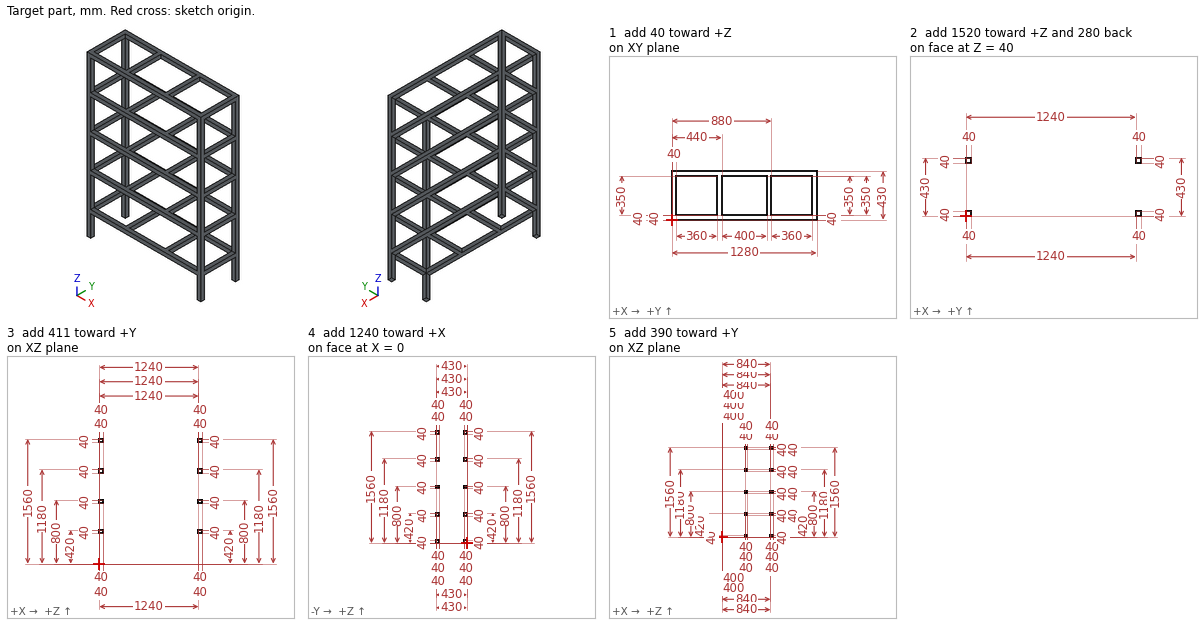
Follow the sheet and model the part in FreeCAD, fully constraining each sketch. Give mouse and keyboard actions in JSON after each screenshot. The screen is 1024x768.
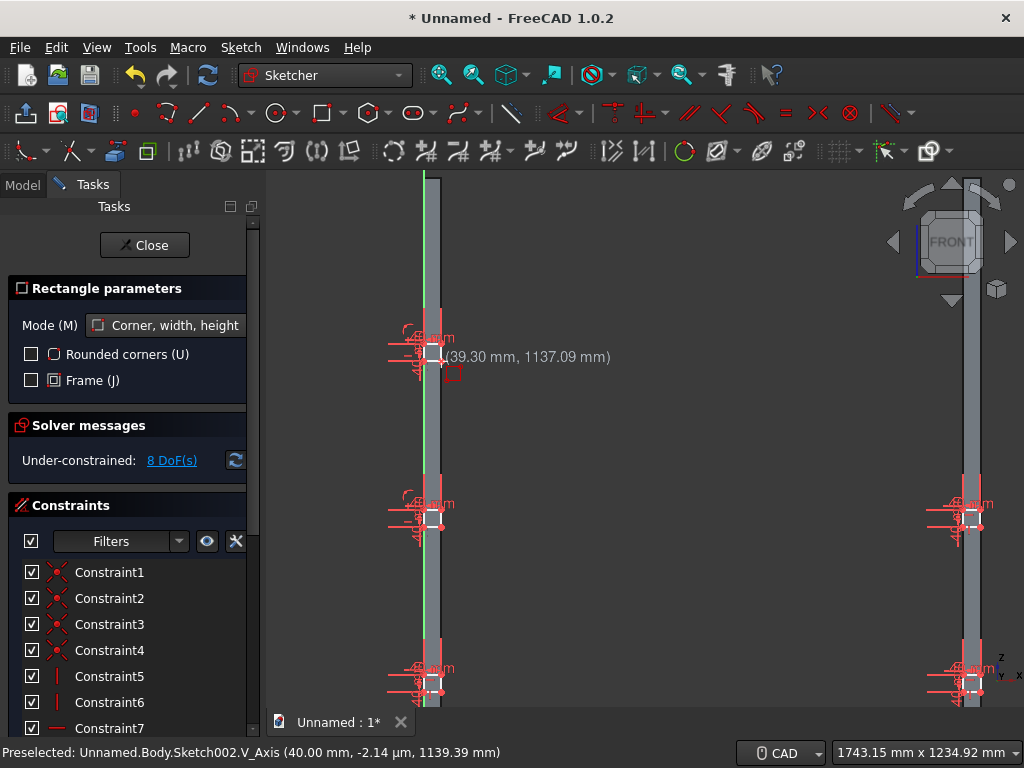
{"action": "scroll", "coordinate": [424, 343], "scroll_direction": "down", "scroll_amount": 3}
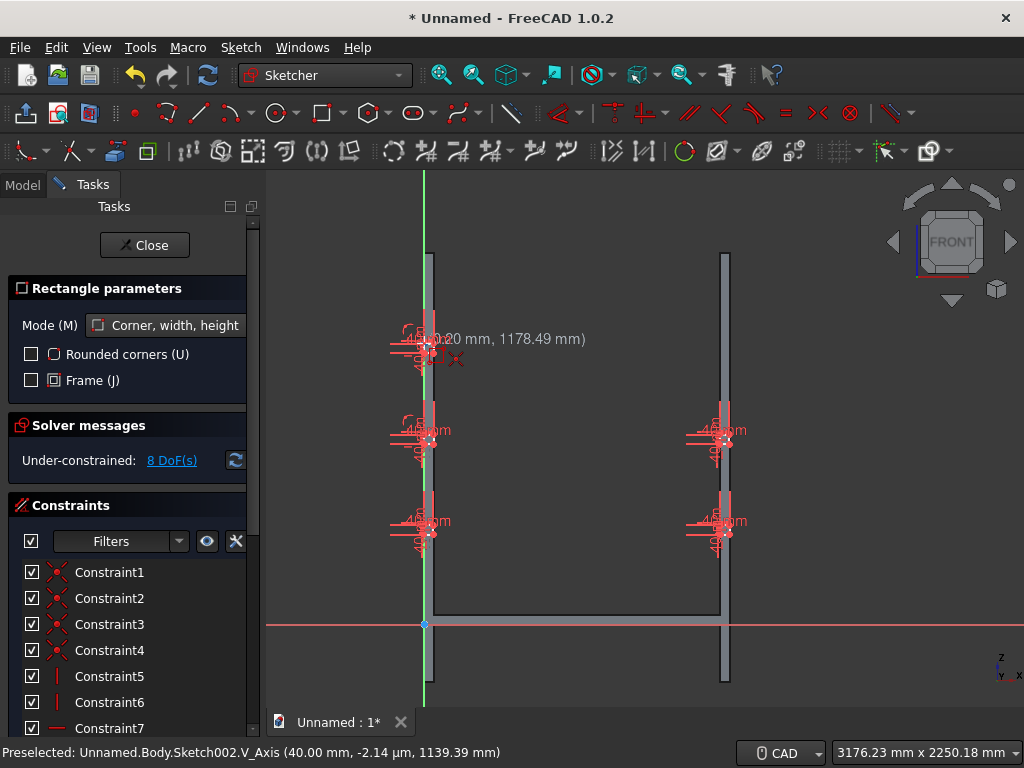
{"action": "scroll", "coordinate": [720, 343], "scroll_direction": "up", "scroll_amount": 3}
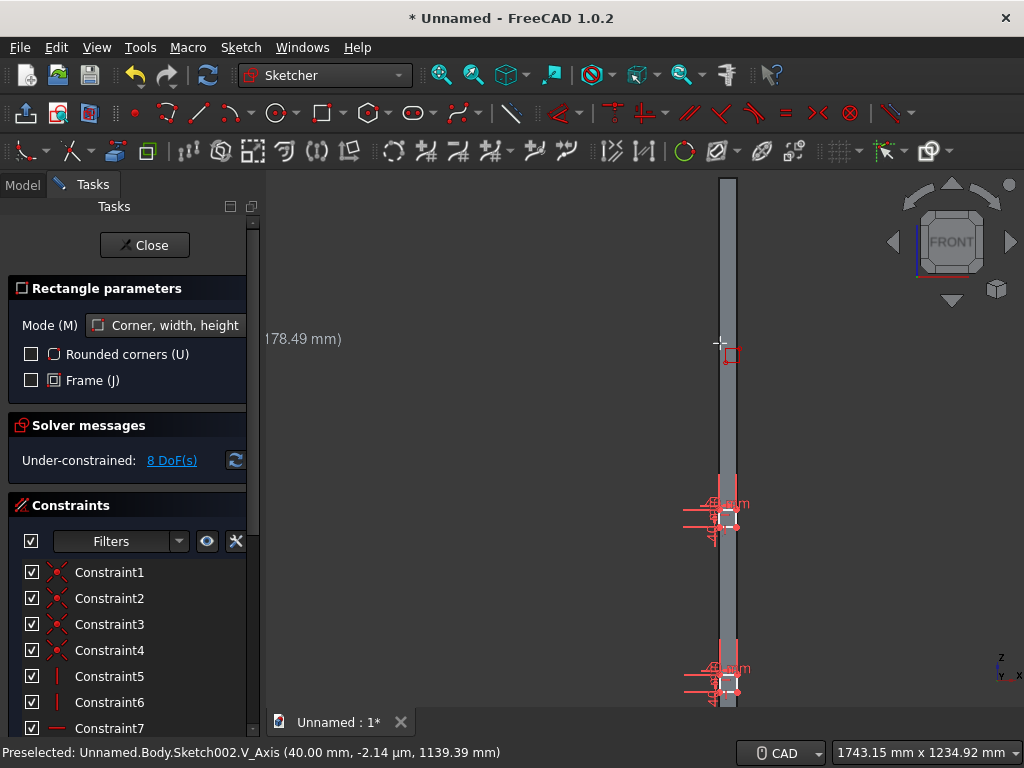
{"action": "left_click", "coordinate": [719, 343]}
{"action": "mouse_move", "coordinate": [737, 361]}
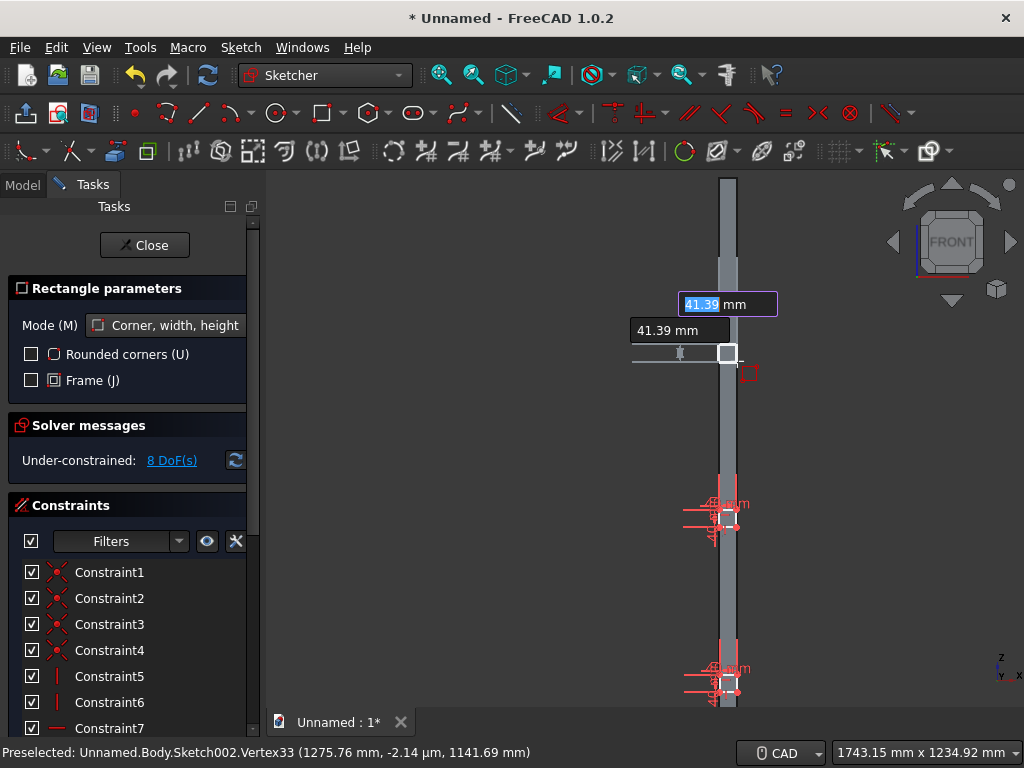
{"action": "type", "text": "40"}
{"action": "key", "text": "Tab"}
{"action": "type", "text": "40"}
{"action": "key", "text": "Return"}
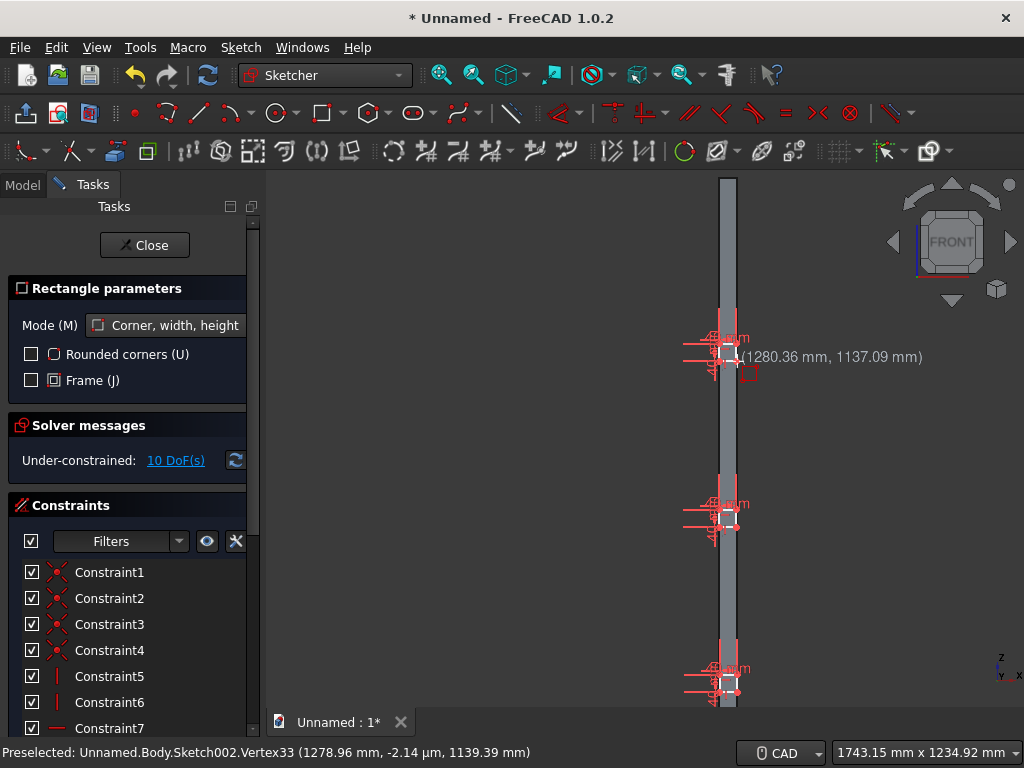
{"action": "scroll", "coordinate": [720, 343], "scroll_direction": "down", "scroll_amount": 3}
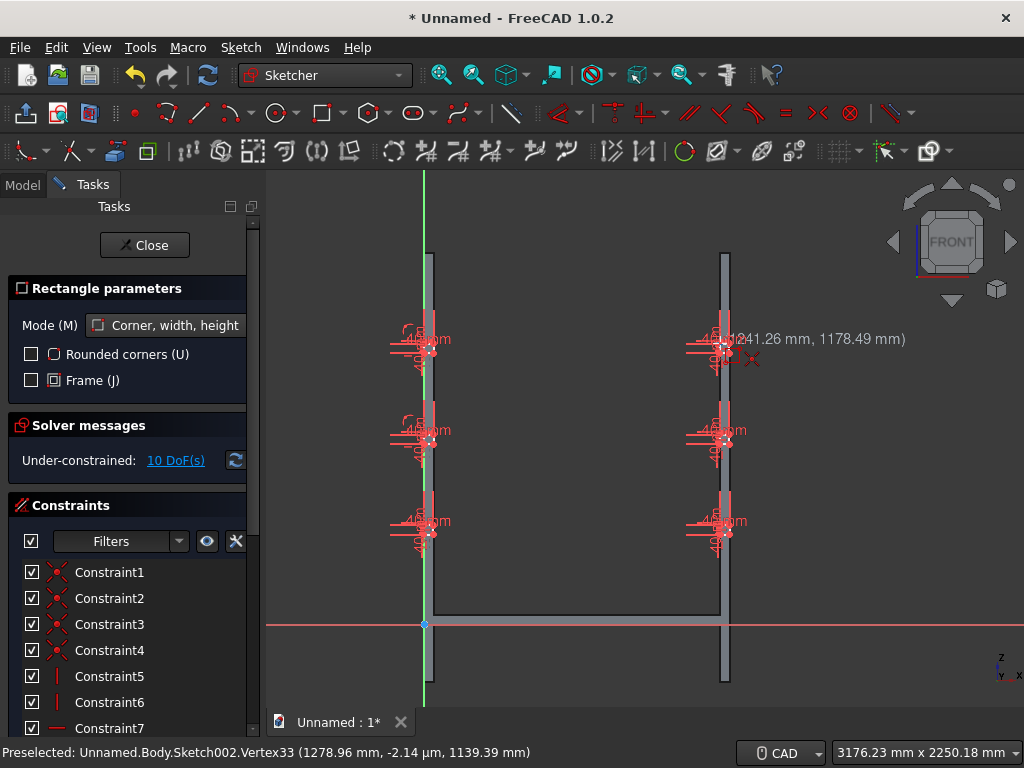
{"action": "scroll", "coordinate": [424, 253], "scroll_direction": "up", "scroll_amount": 3}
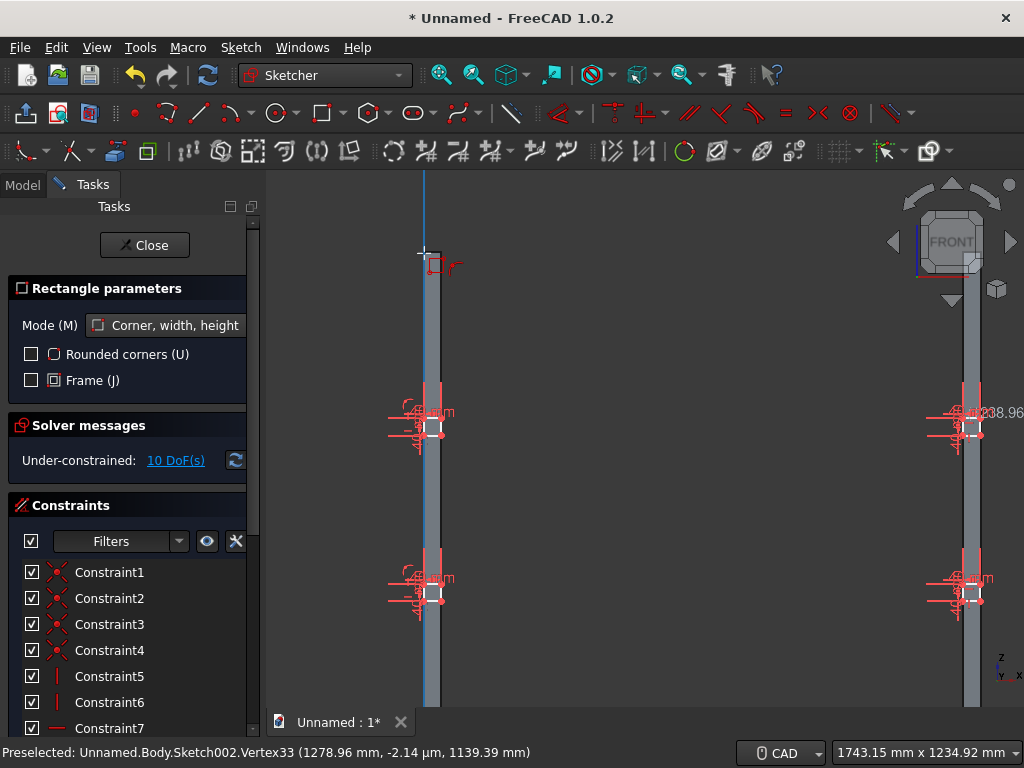
{"action": "left_click", "coordinate": [424, 252]}
{"action": "mouse_move", "coordinate": [441, 270]}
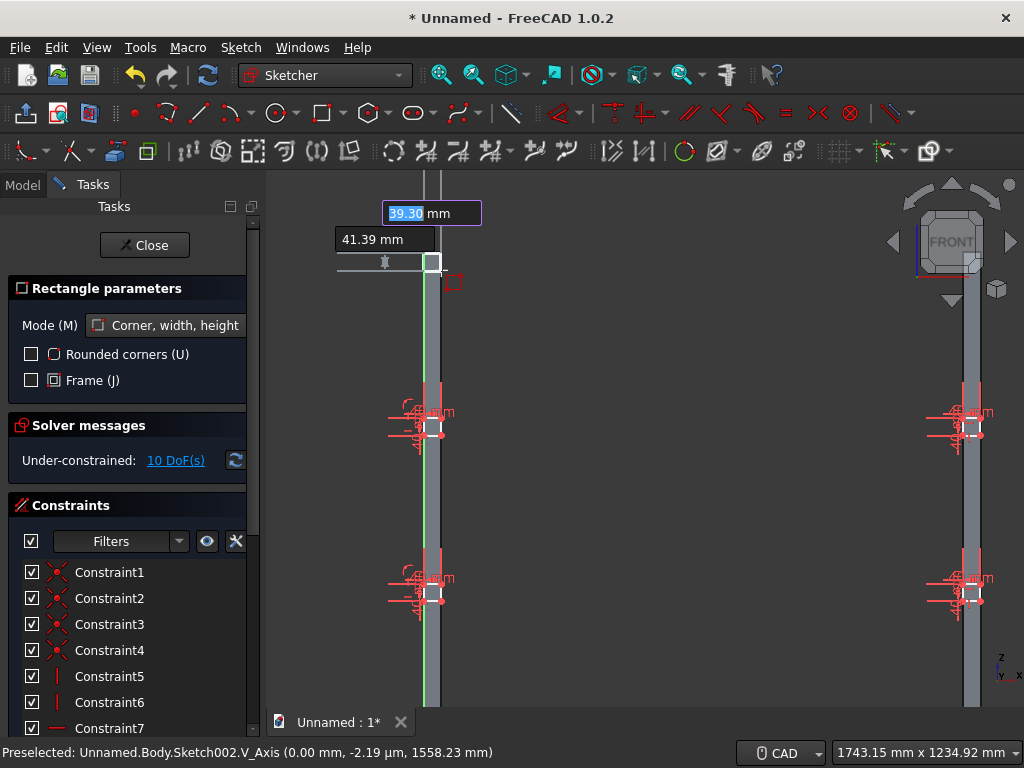
{"action": "type", "text": "40"}
{"action": "key", "text": "Tab"}
{"action": "type", "text": "40"}
{"action": "key", "text": "Return"}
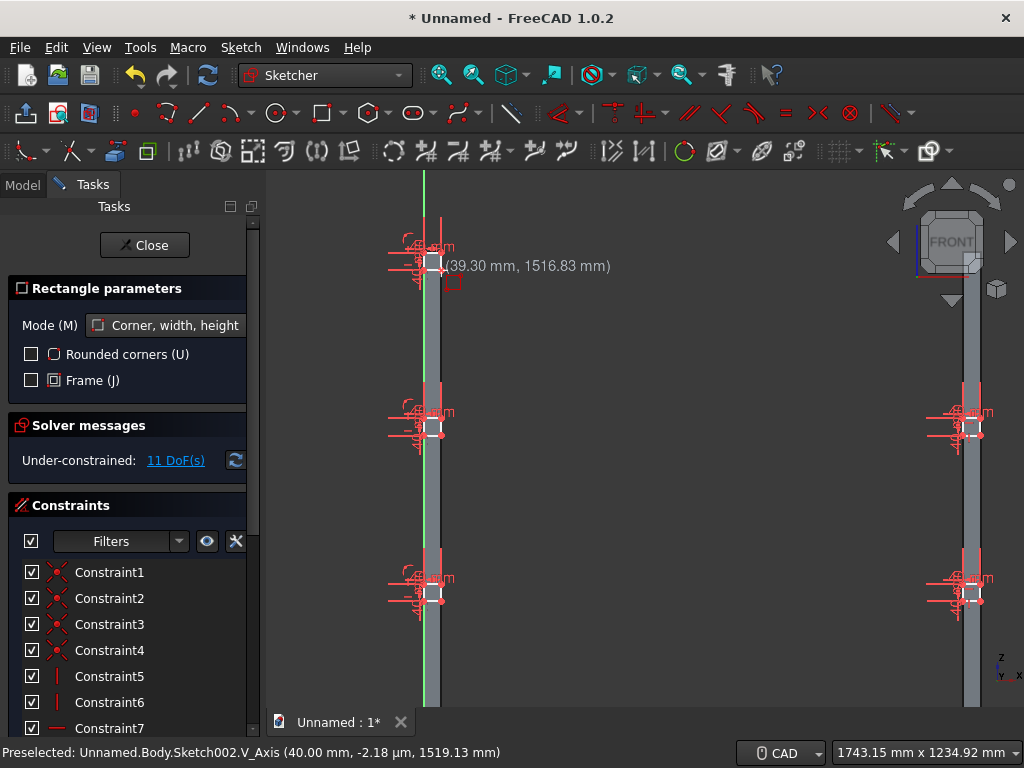
{"action": "scroll", "coordinate": [424, 253], "scroll_direction": "down", "scroll_amount": 3}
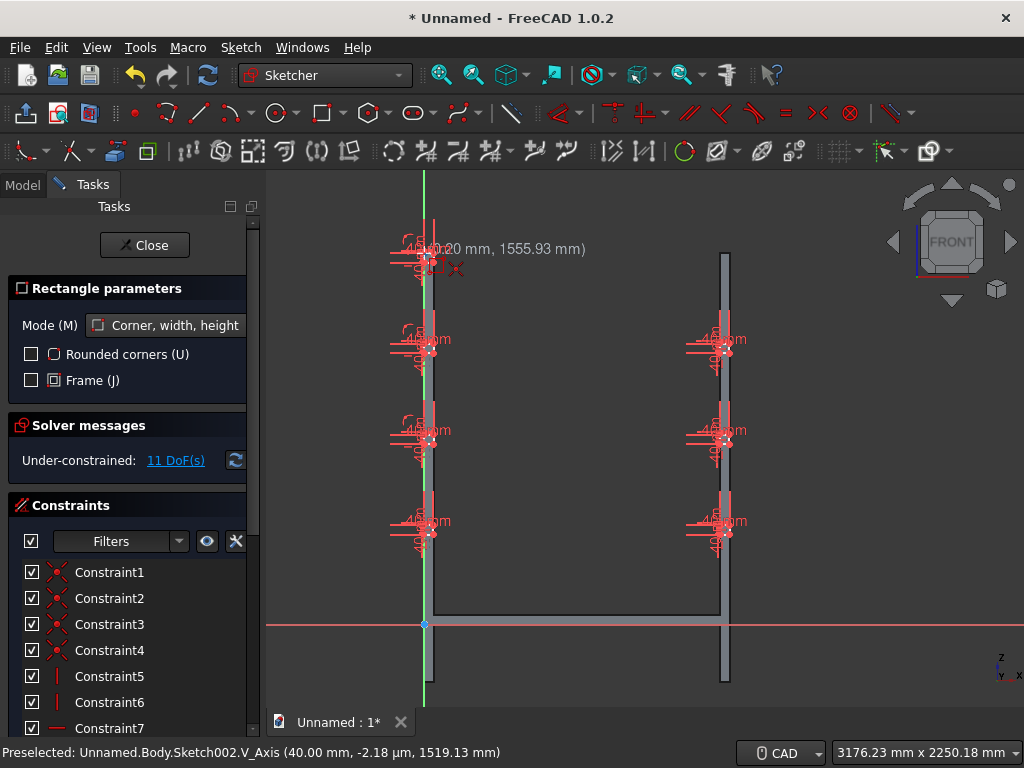
{"action": "scroll", "coordinate": [720, 253], "scroll_direction": "up", "scroll_amount": 3}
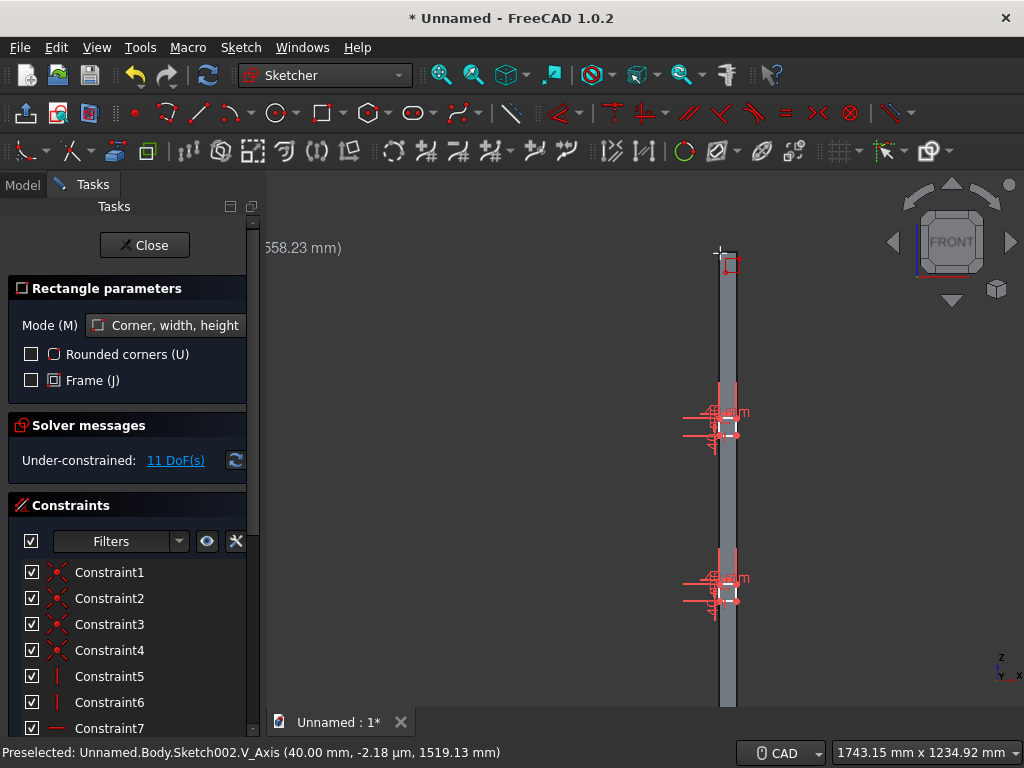
{"action": "left_click", "coordinate": [719, 252]}
{"action": "mouse_move", "coordinate": [737, 270]}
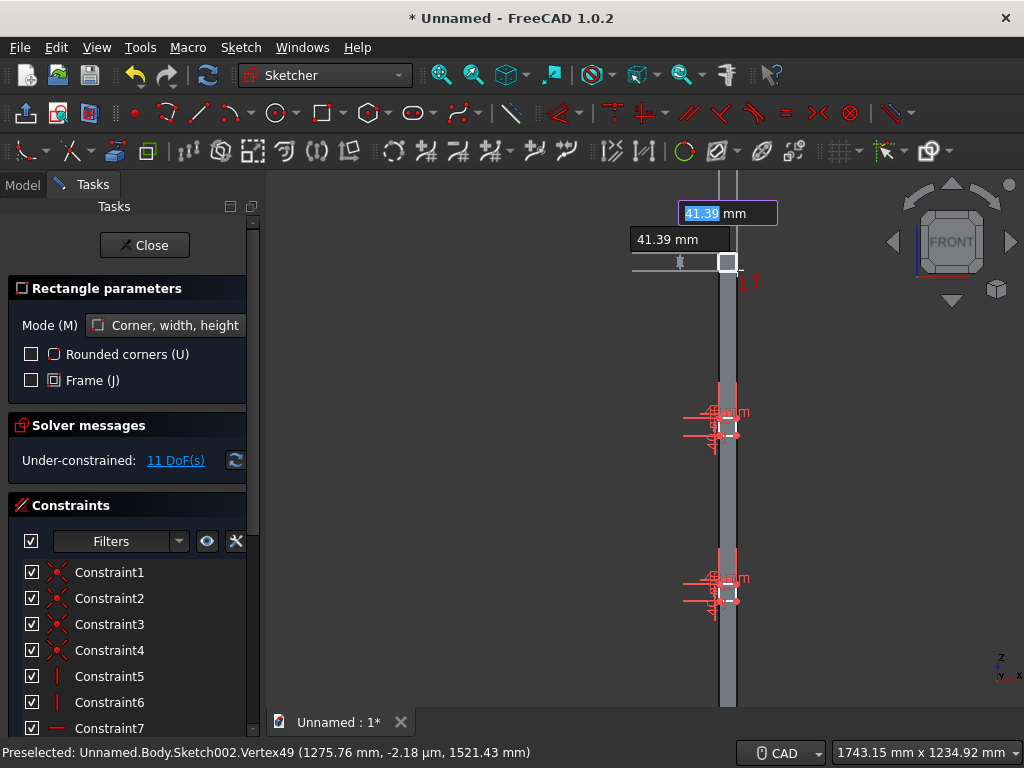
{"action": "type", "text": "40"}
{"action": "key", "text": "Tab"}
{"action": "type", "text": "40"}
{"action": "key", "text": "Return"}
{"action": "key", "text": "Escape"}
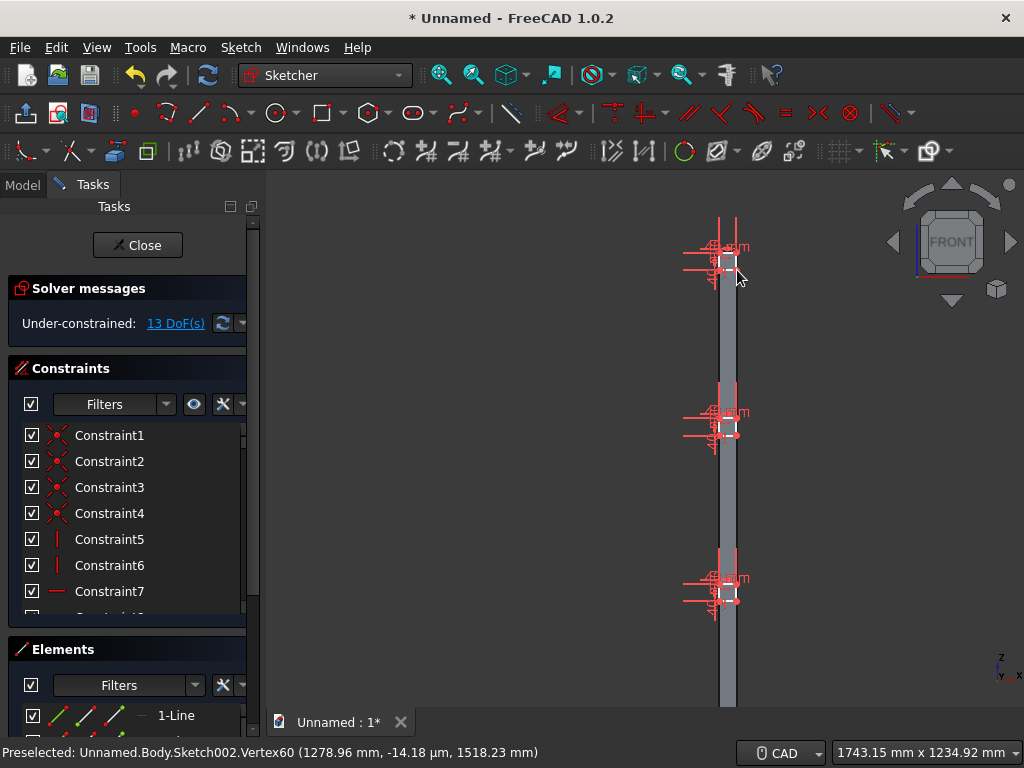
{"action": "scroll", "coordinate": [720, 253], "scroll_direction": "down", "scroll_amount": 3}